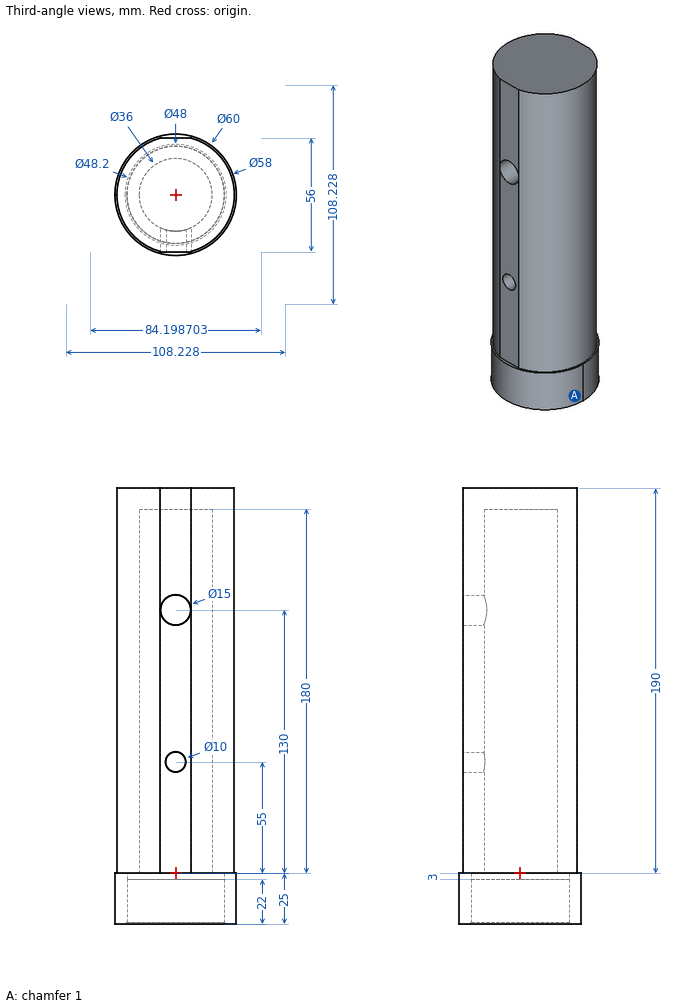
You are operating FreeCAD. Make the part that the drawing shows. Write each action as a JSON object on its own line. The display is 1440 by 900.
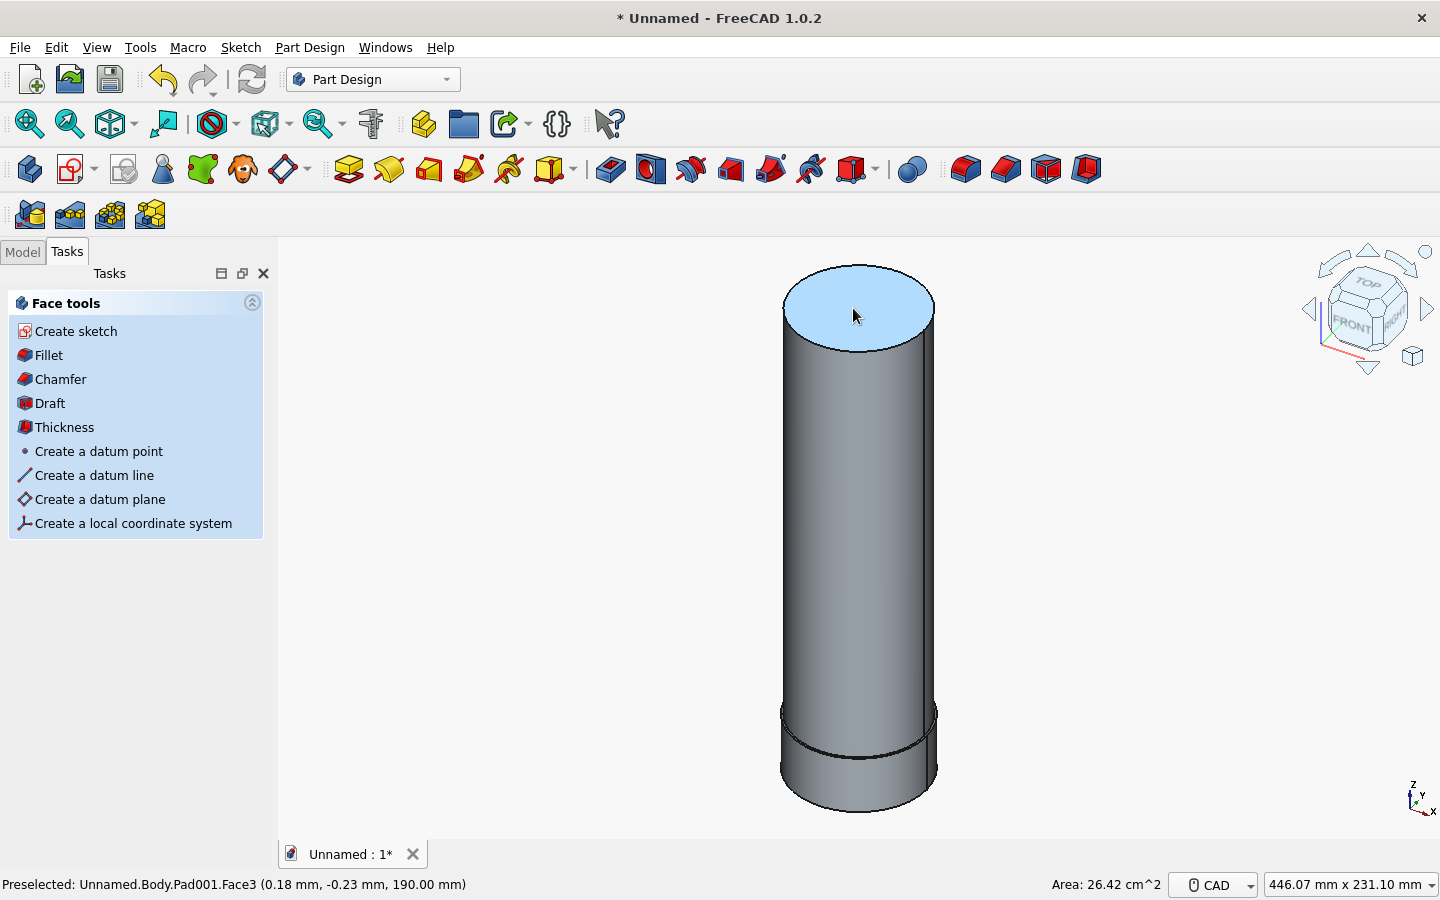
{"action": "left_click", "coordinate": [70, 170]}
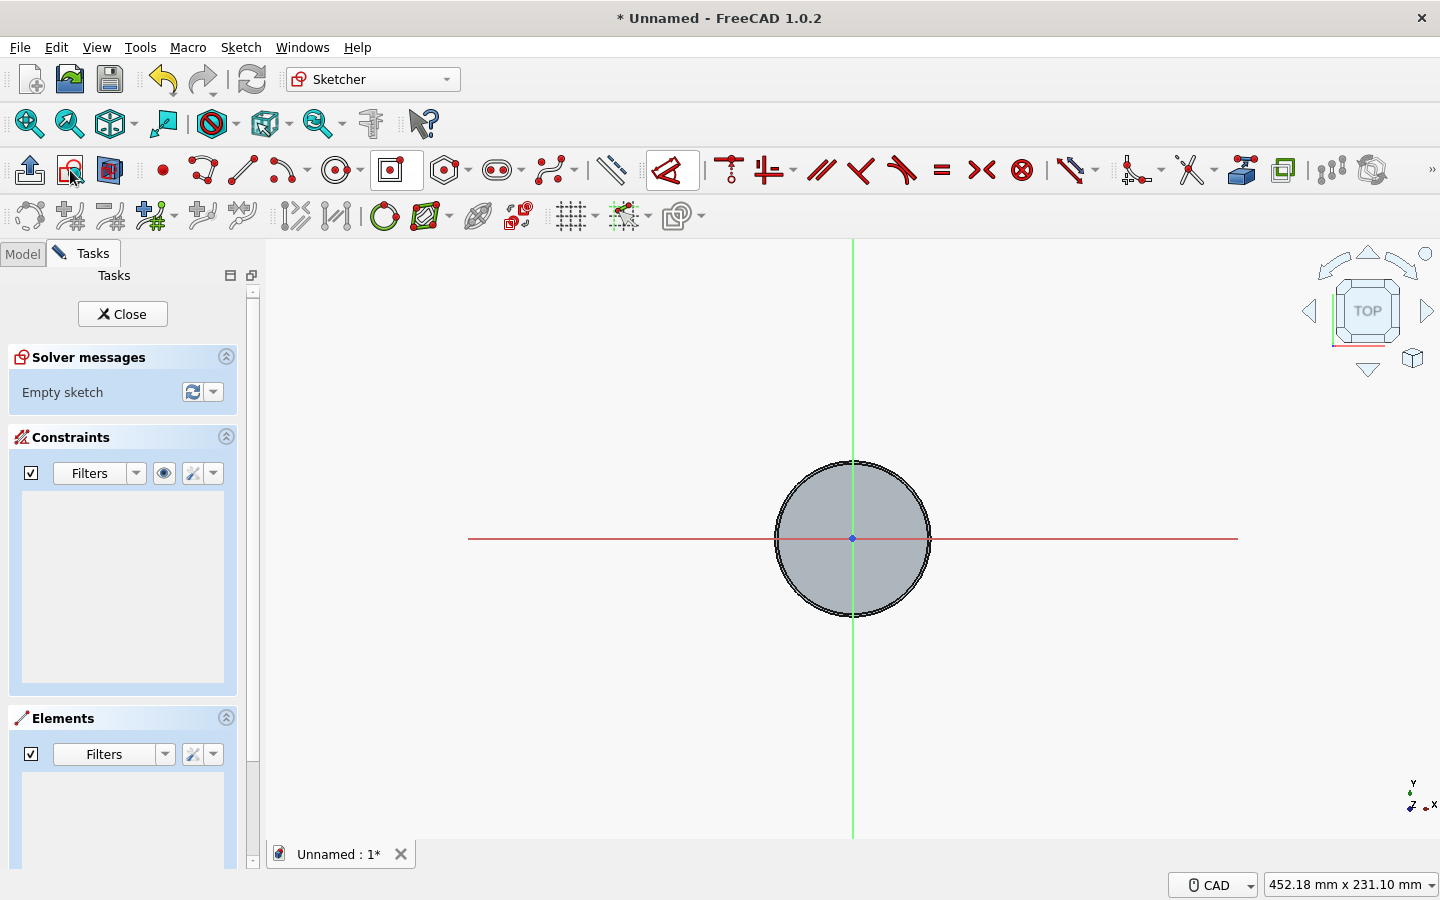
{"action": "scroll", "coordinate": [992, 539], "scroll_direction": "up", "scroll_amount": 2}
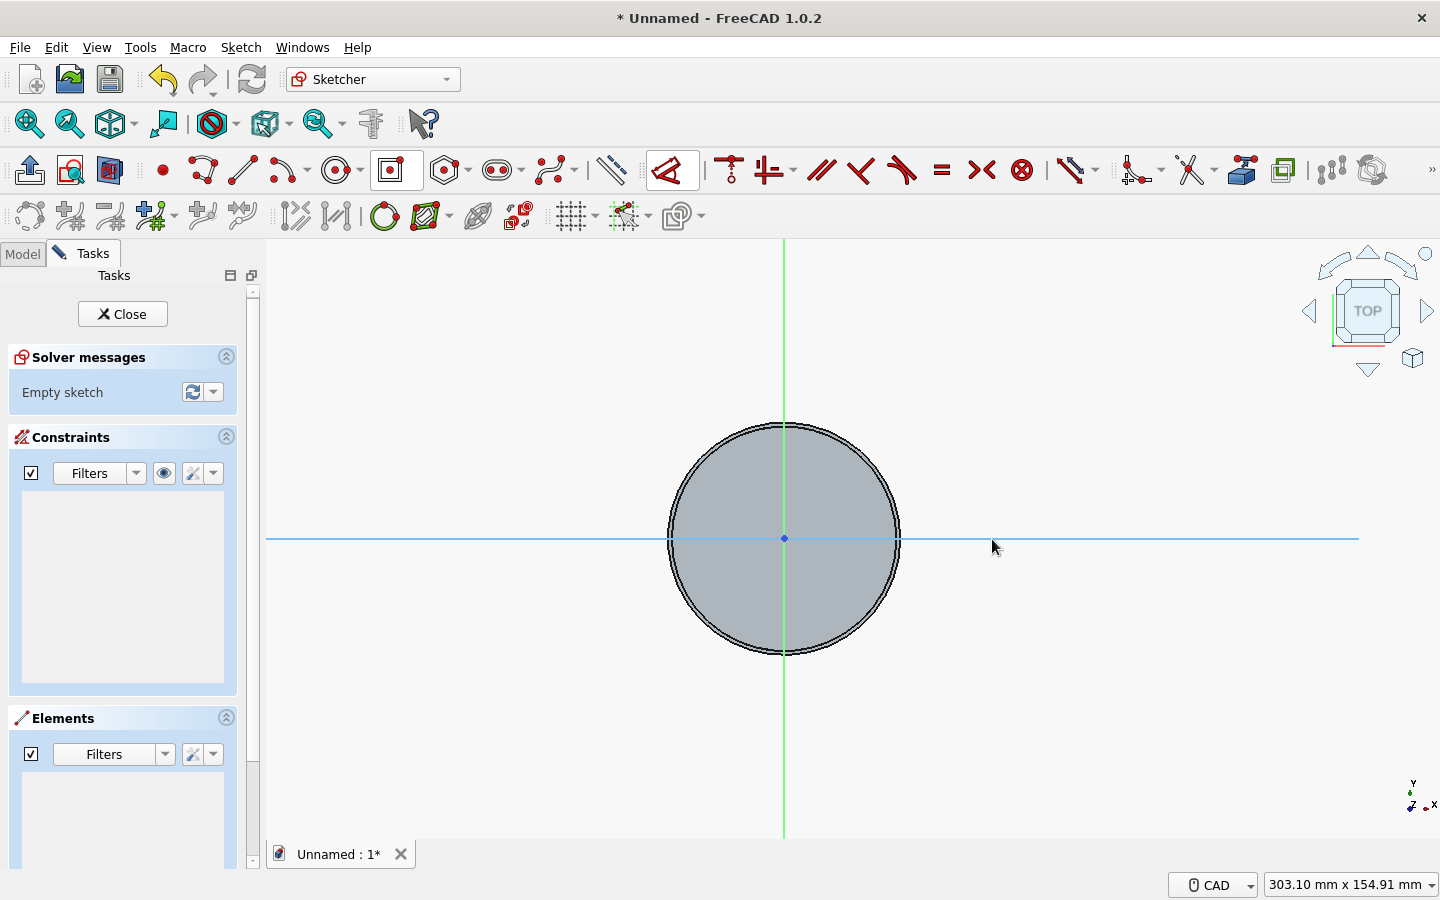
{"action": "left_click", "coordinate": [390, 170]}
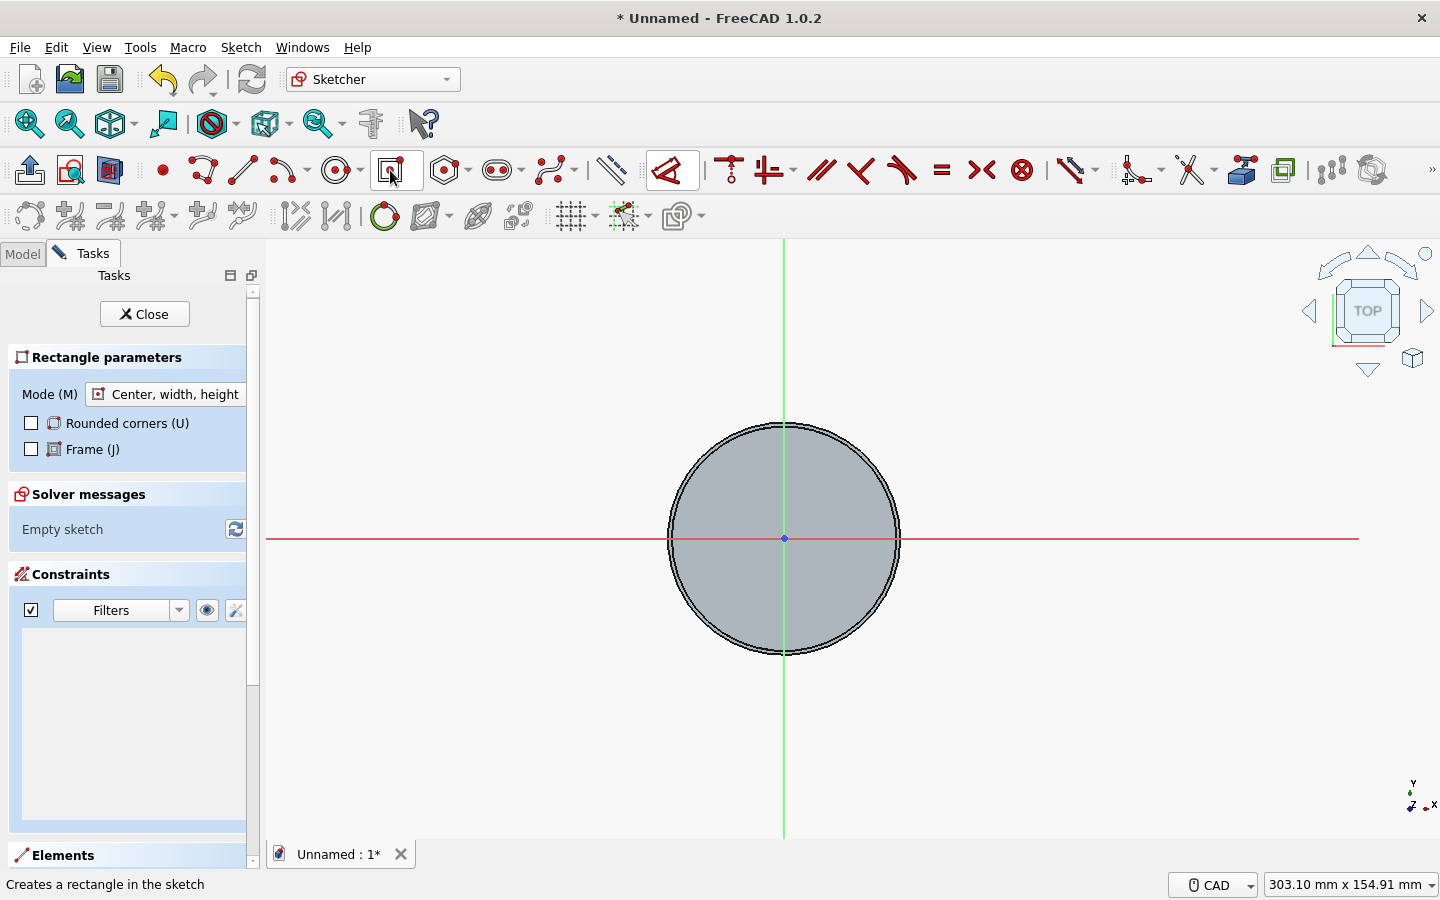
{"action": "left_click", "coordinate": [784, 539]}
{"action": "left_click", "coordinate": [994, 329]}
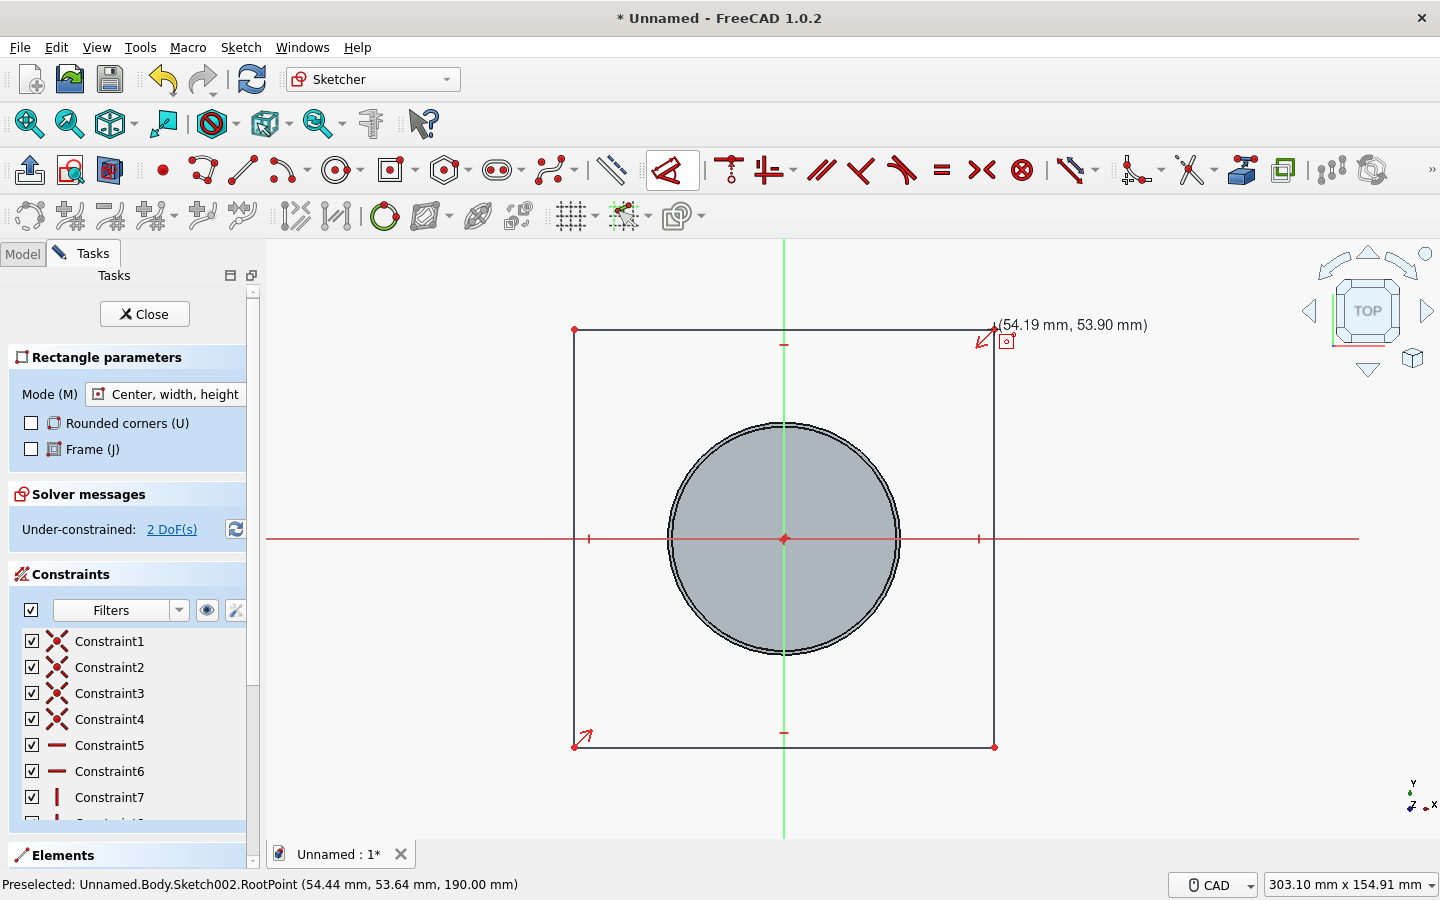
{"action": "left_click", "coordinate": [784, 539]}
{"action": "left_click", "coordinate": [947, 430]}
{"action": "key", "text": "Escape"}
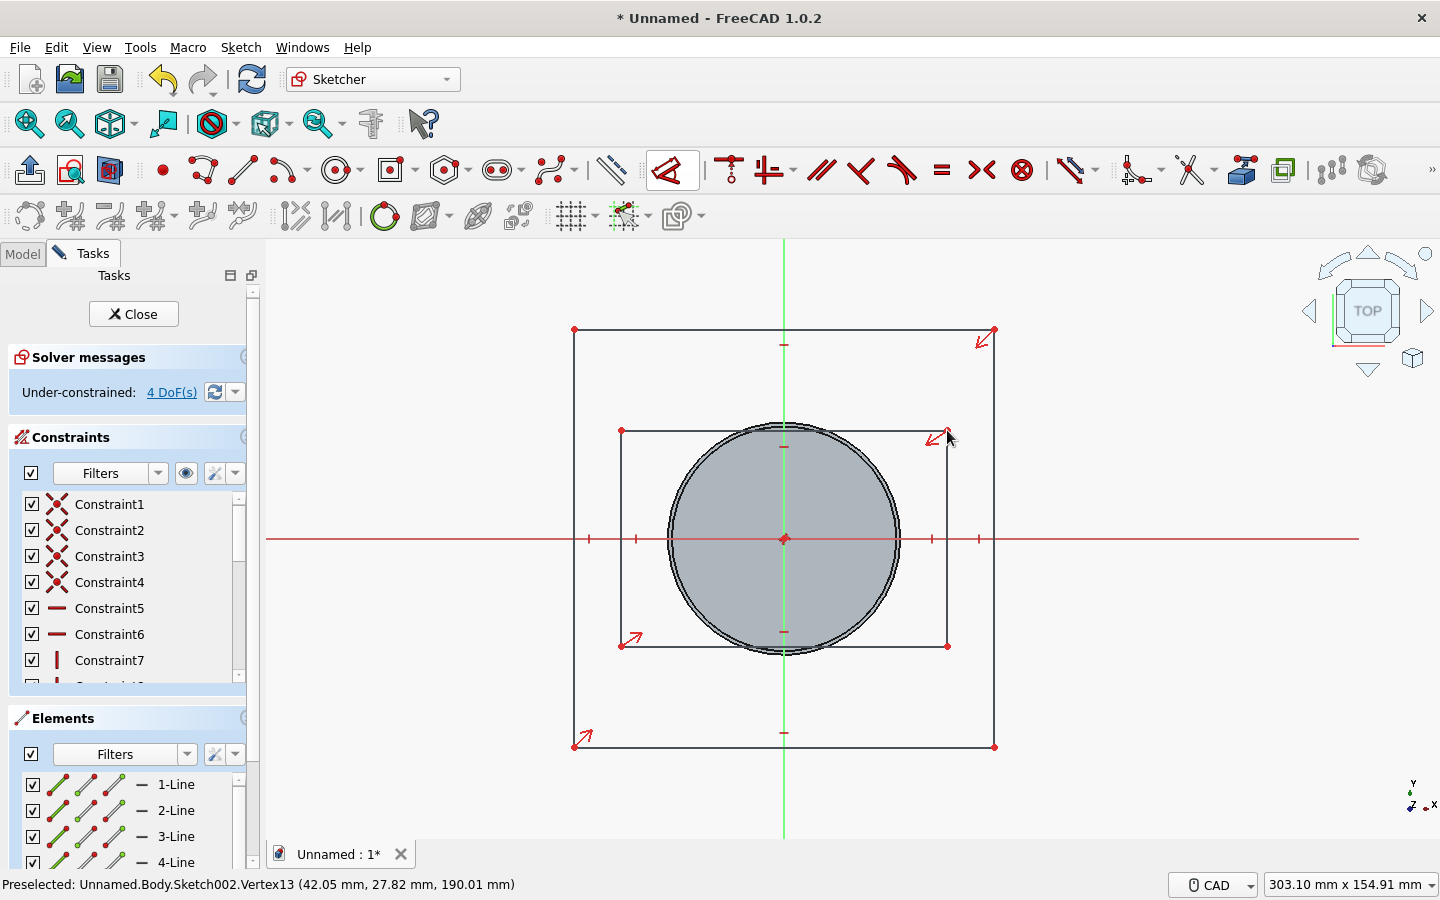
{"action": "left_click", "coordinate": [947, 582]}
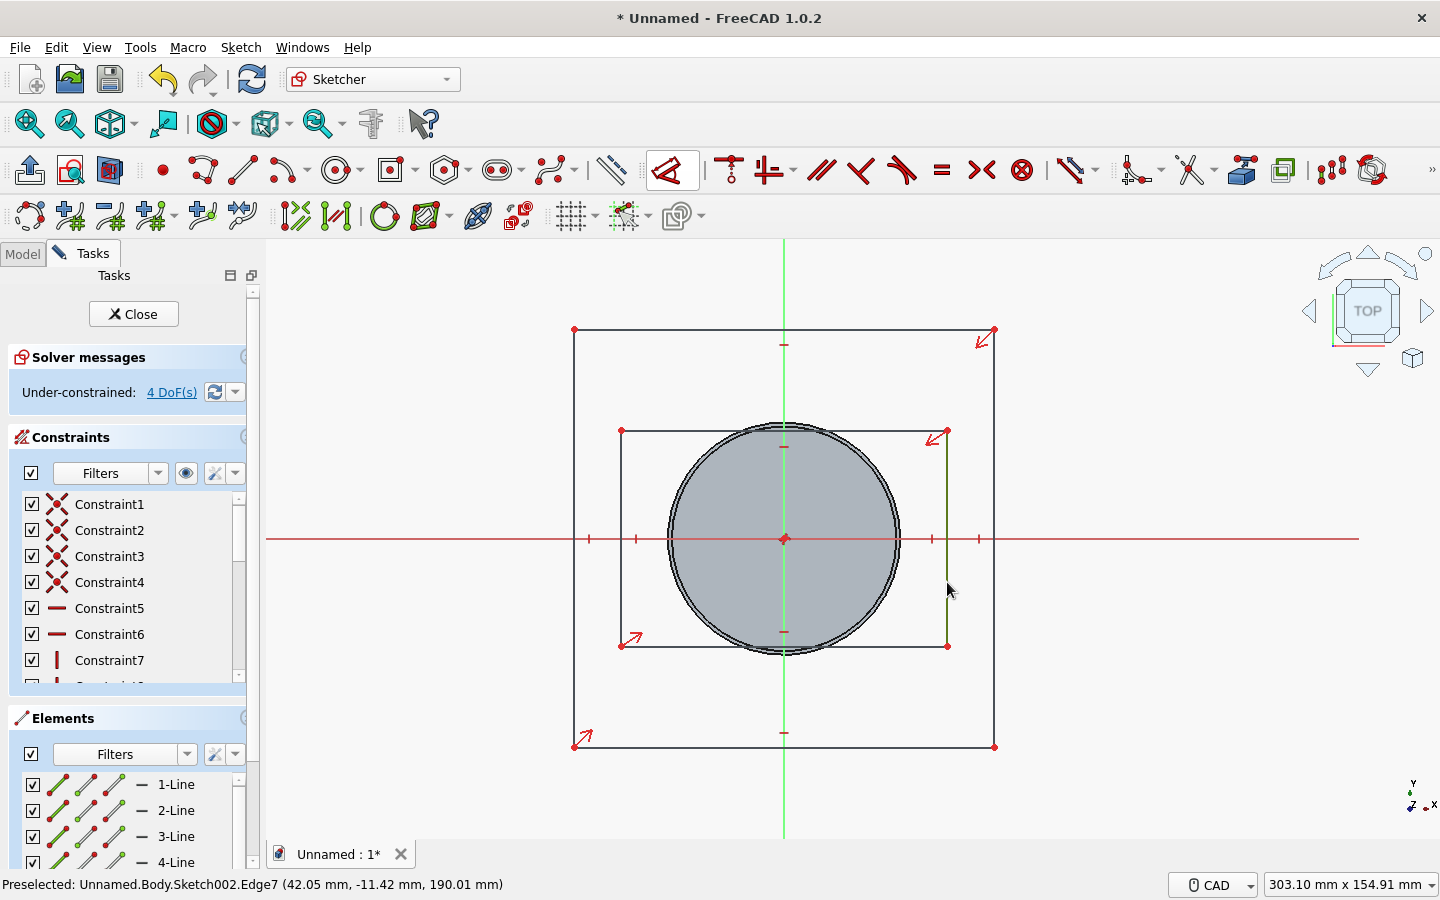
{"action": "left_click", "coordinate": [694, 170]}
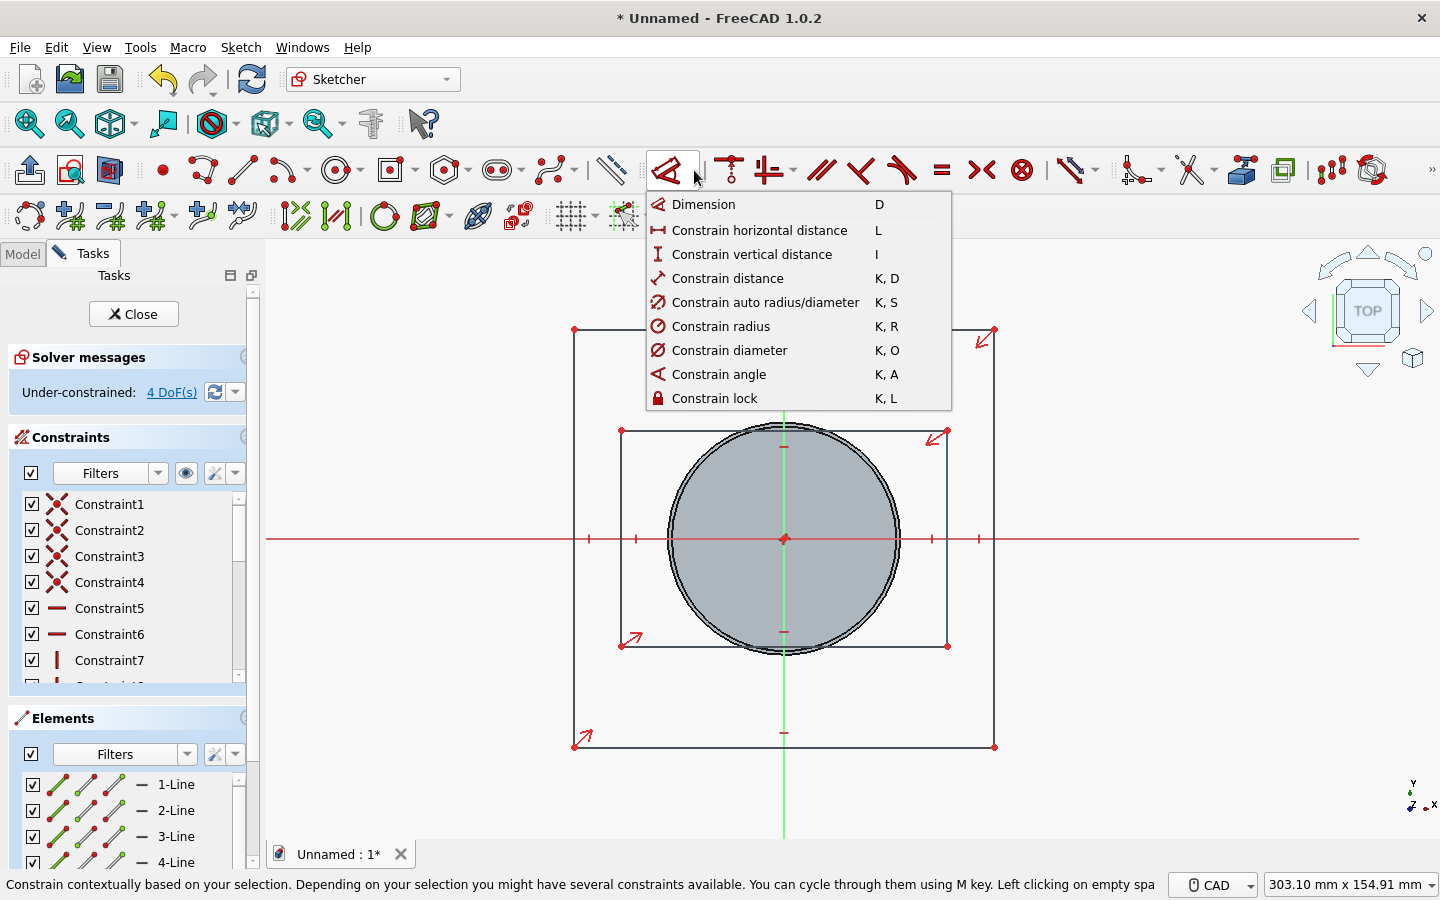
{"action": "left_click", "coordinate": [799, 254]}